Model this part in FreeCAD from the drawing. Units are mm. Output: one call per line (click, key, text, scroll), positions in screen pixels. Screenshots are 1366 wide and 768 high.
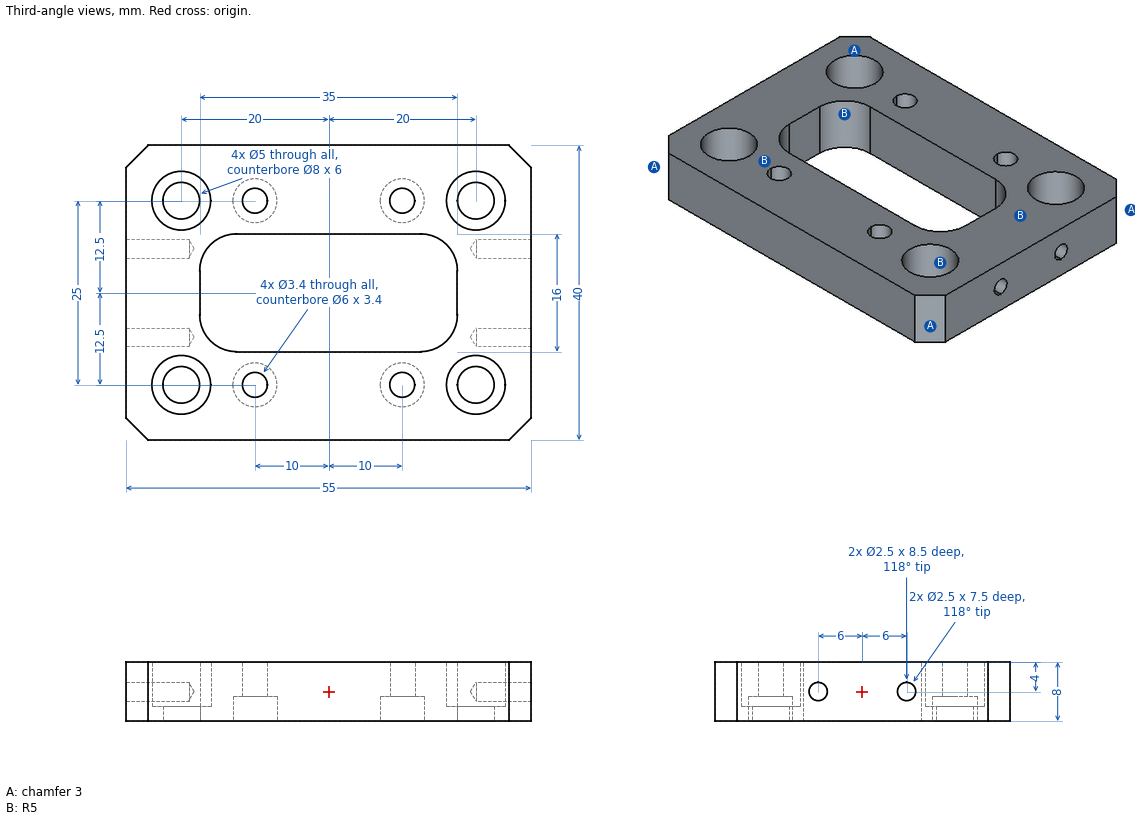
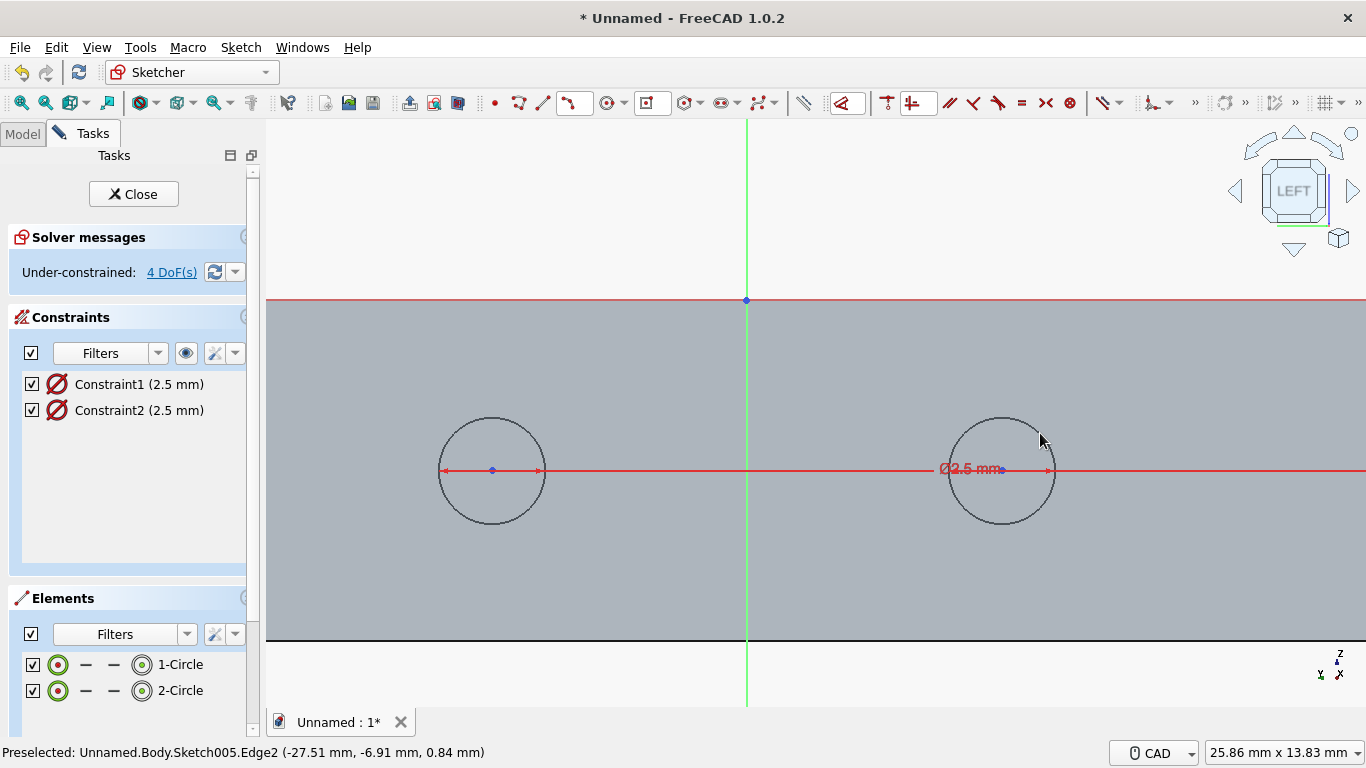
click(492, 471)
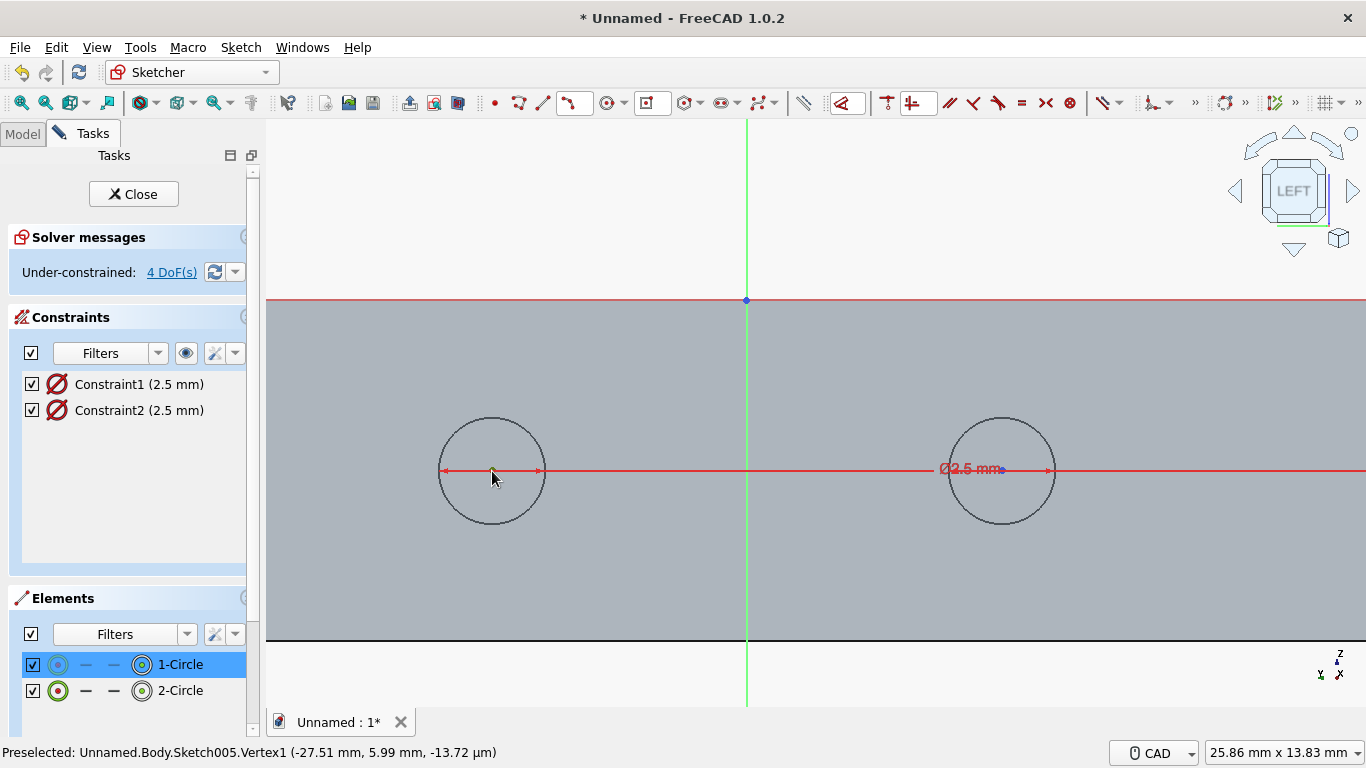
click(1002, 471)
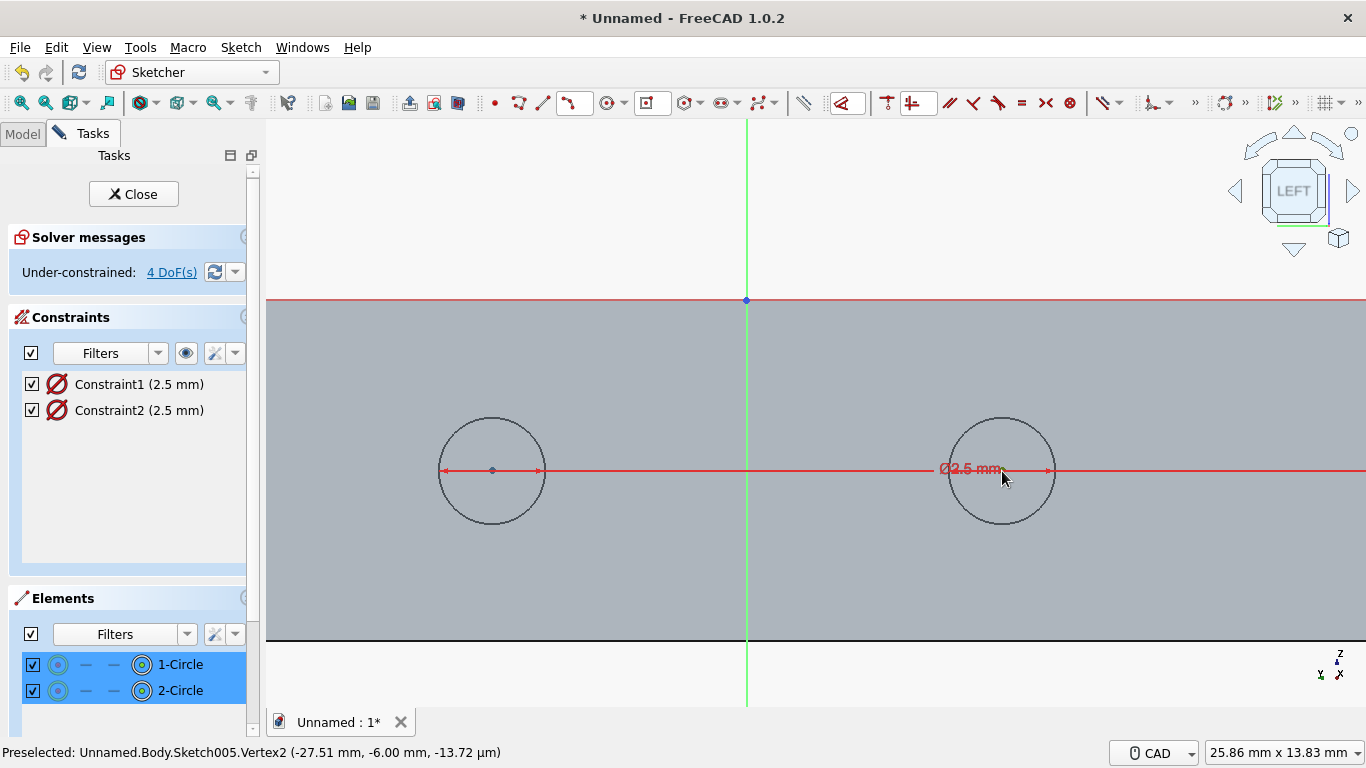
click(932, 104)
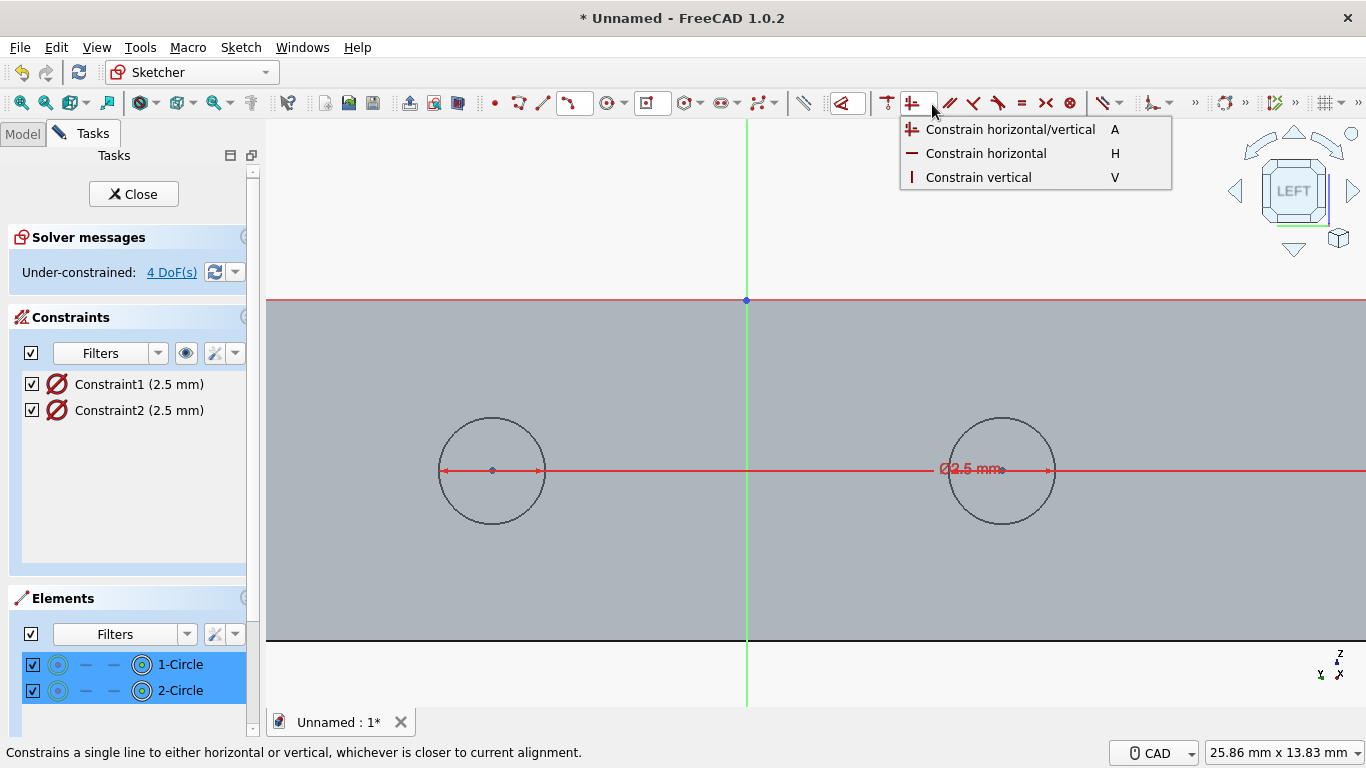
click(1036, 153)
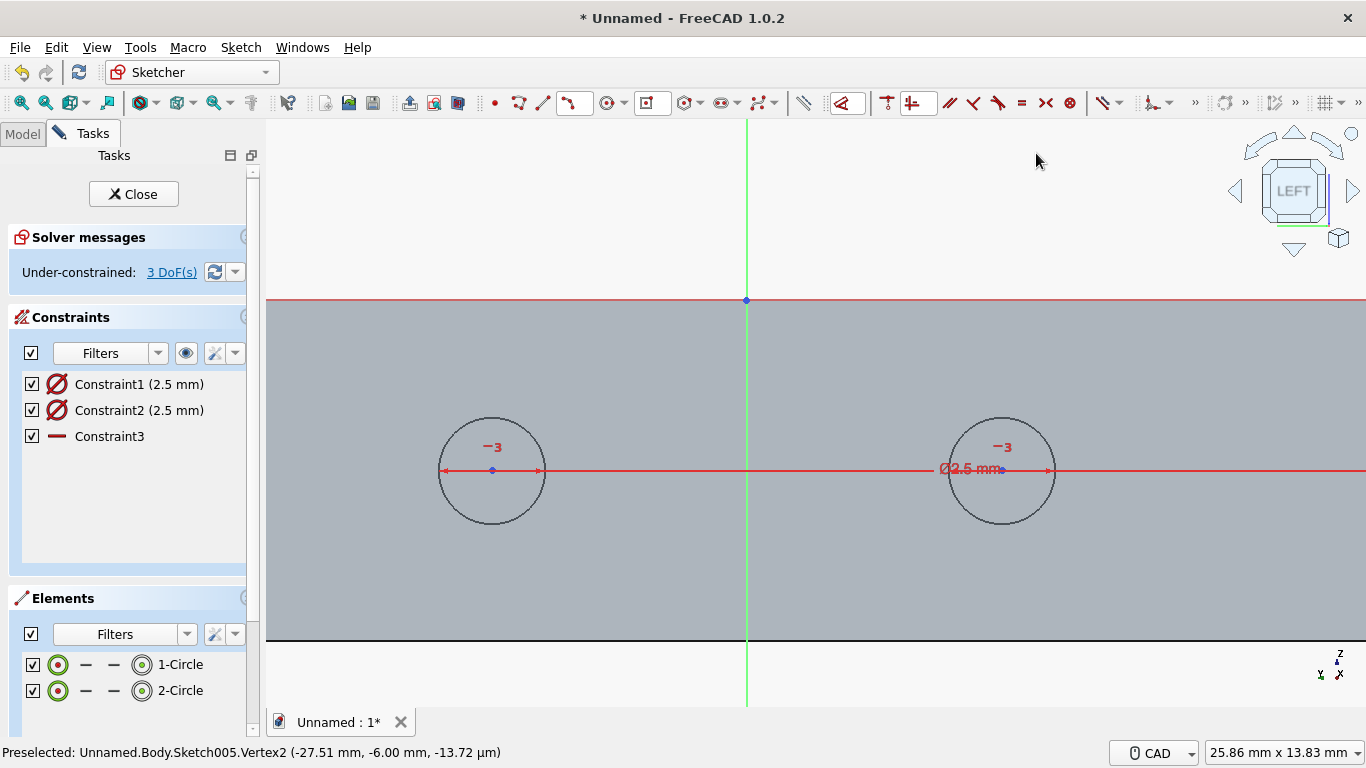
click(492, 471)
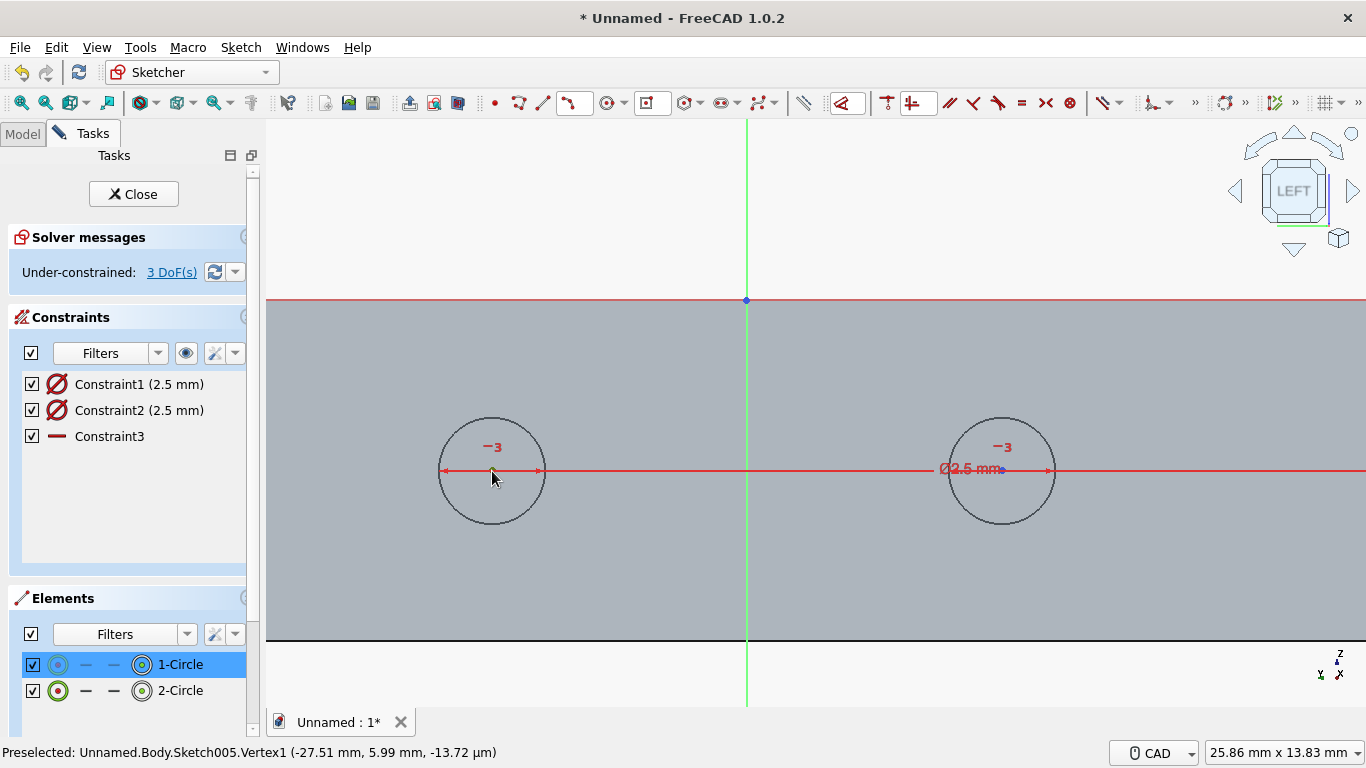
click(860, 104)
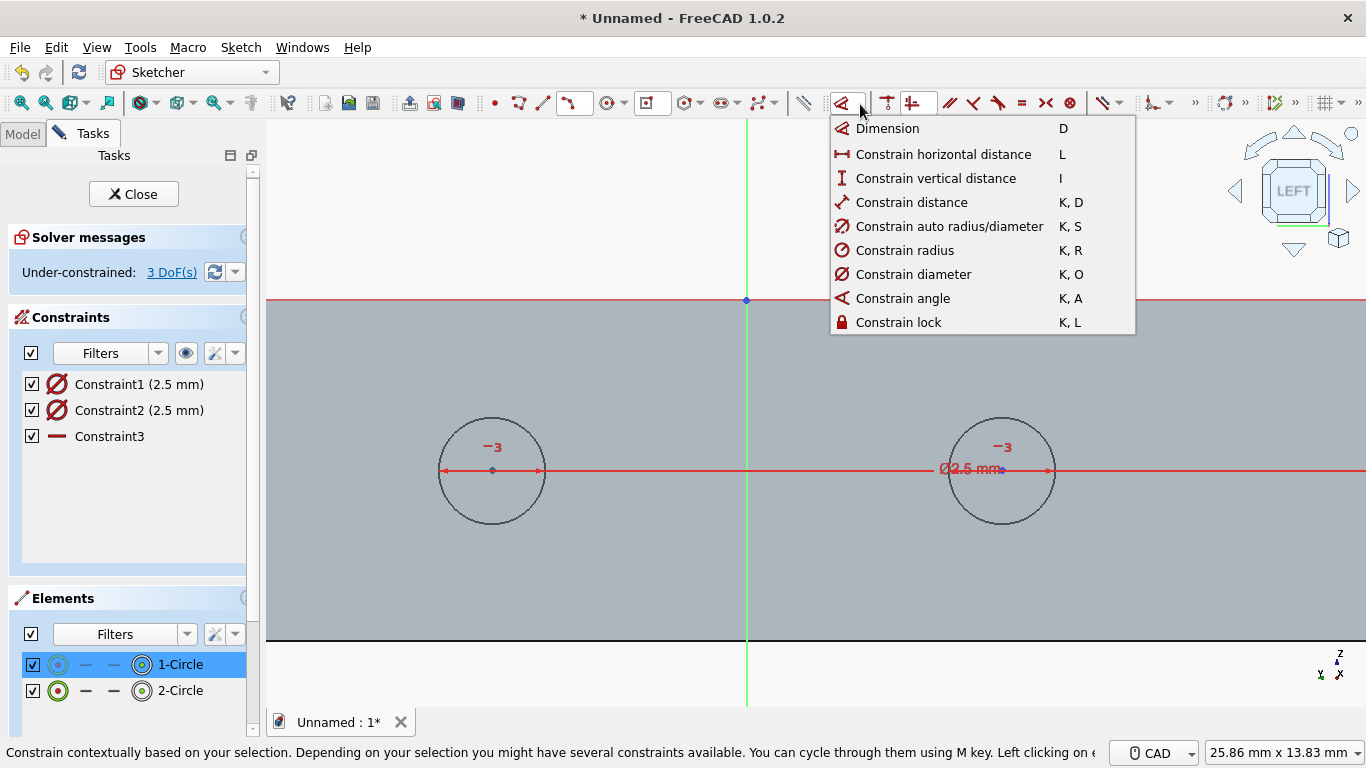
click(983, 154)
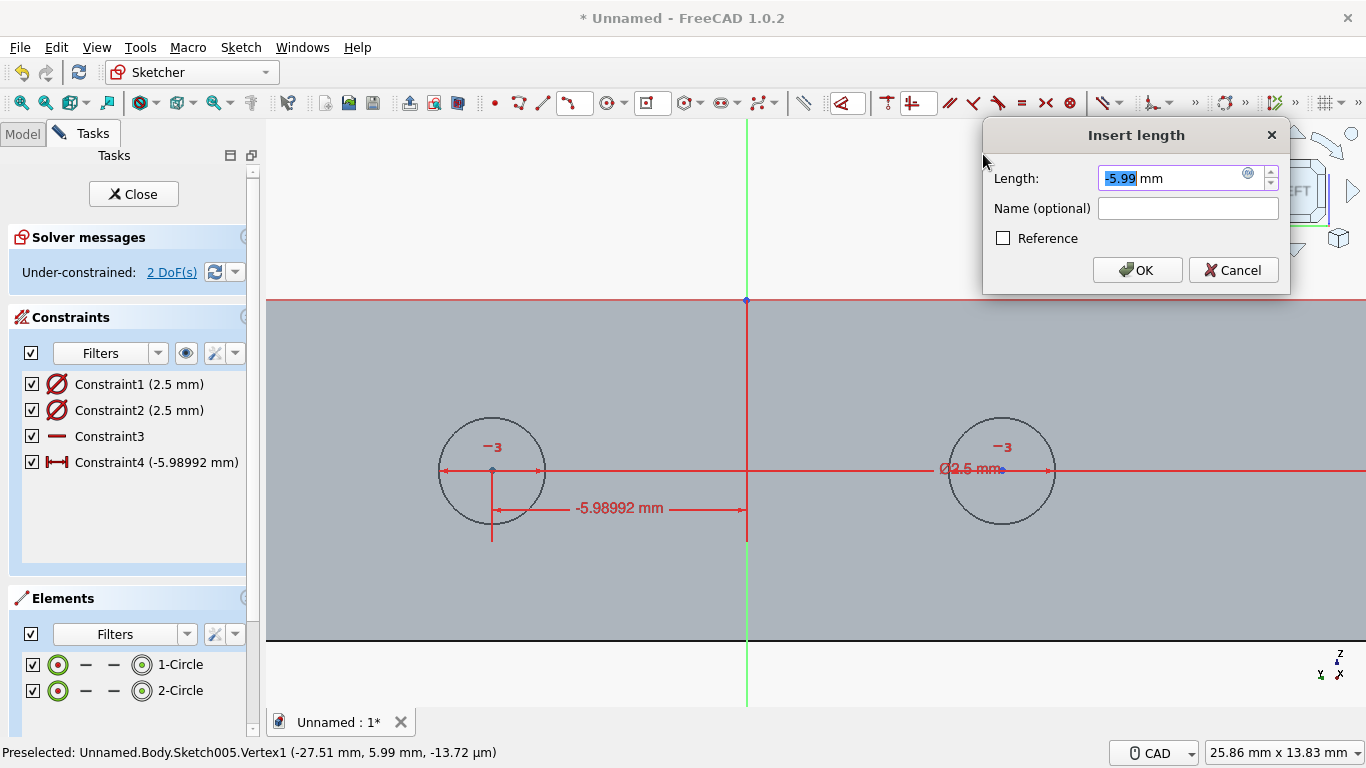
text(-6)
key(Return)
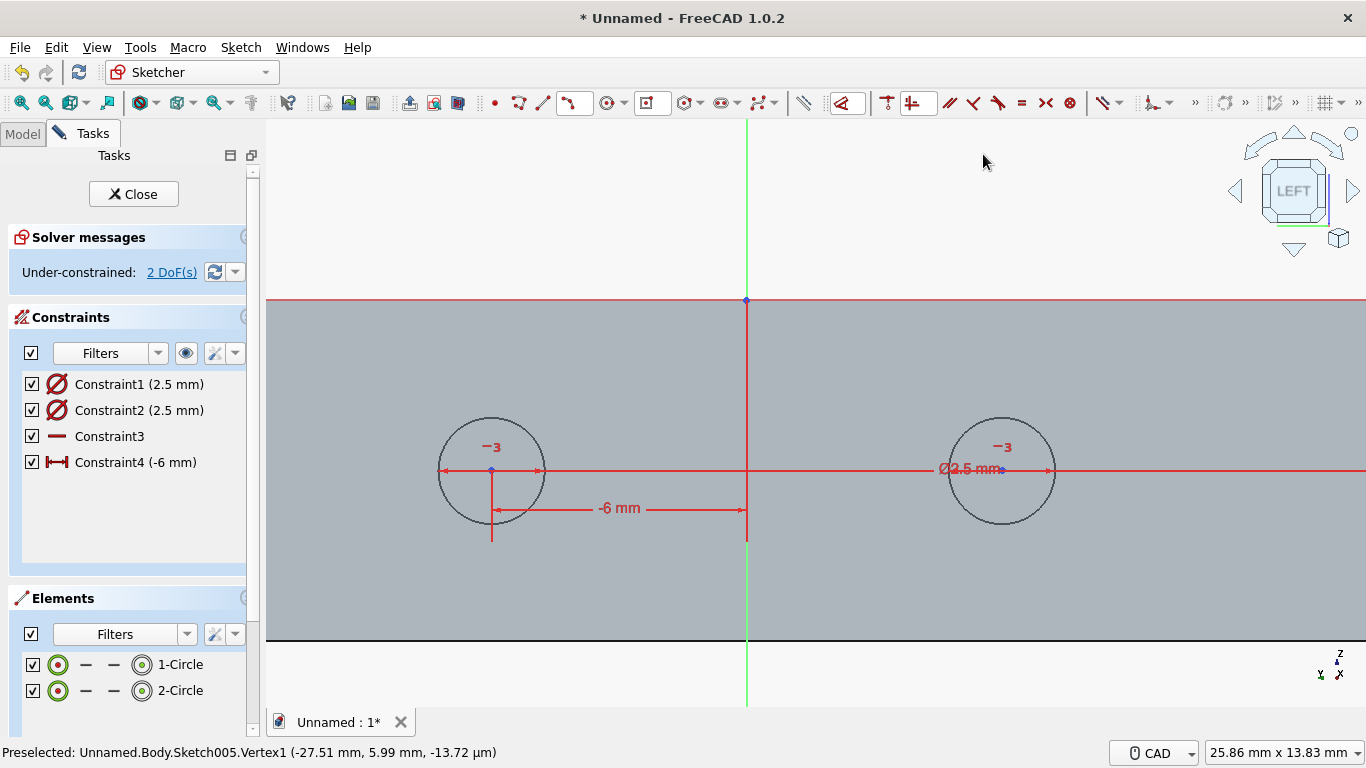
click(492, 471)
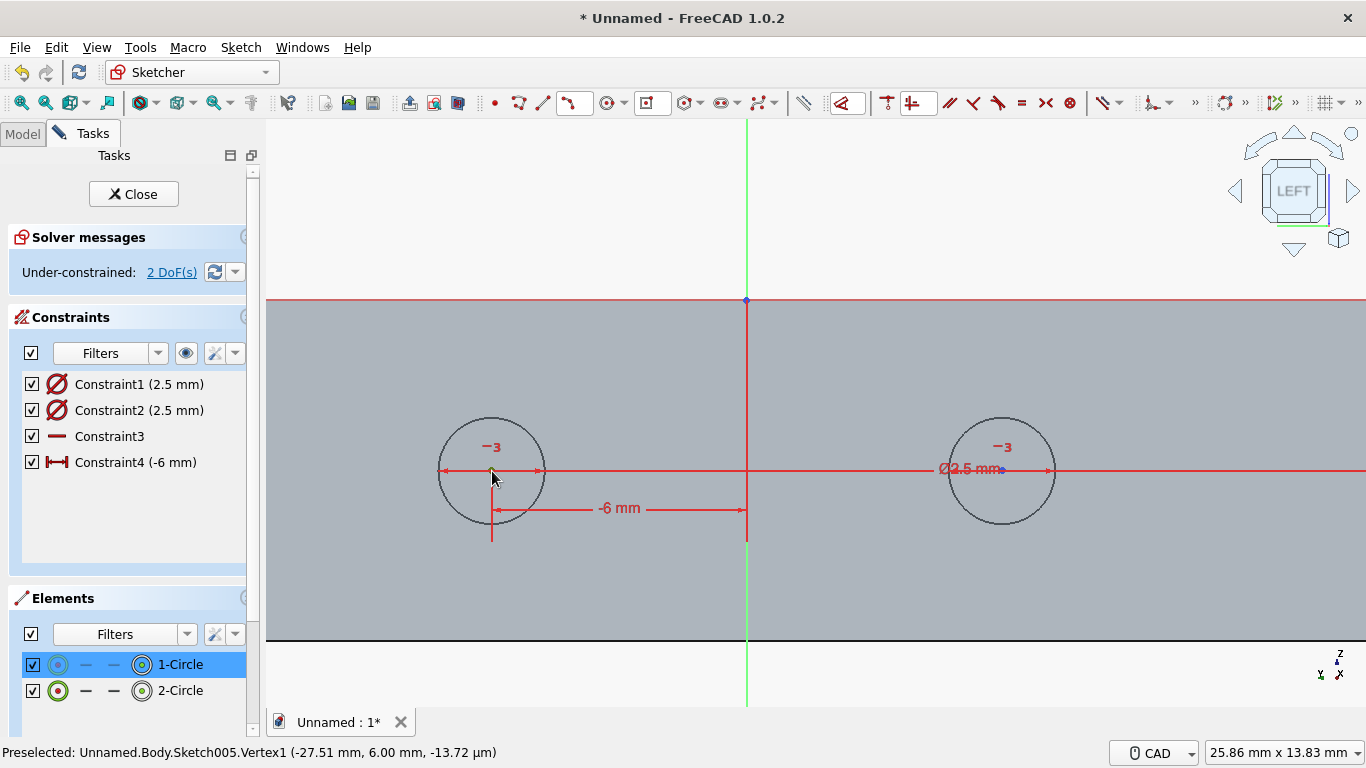
click(860, 104)